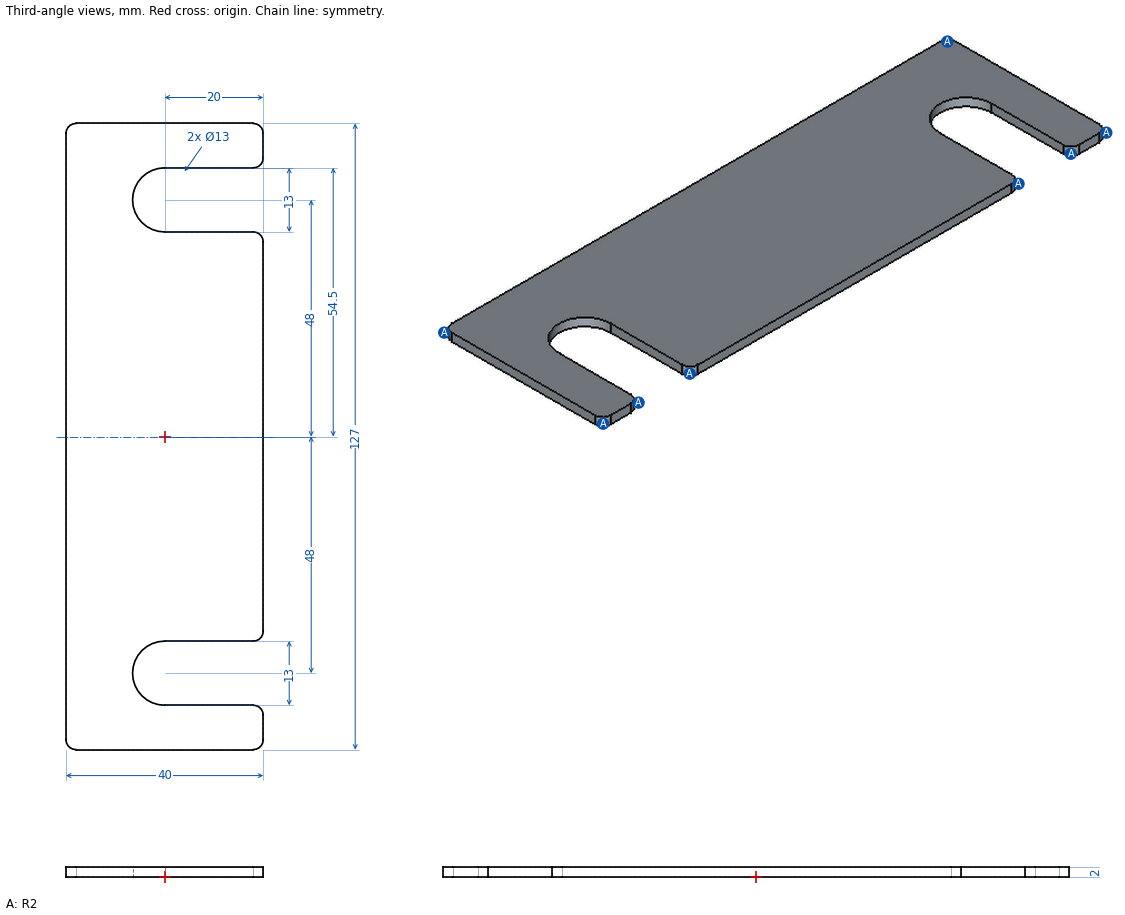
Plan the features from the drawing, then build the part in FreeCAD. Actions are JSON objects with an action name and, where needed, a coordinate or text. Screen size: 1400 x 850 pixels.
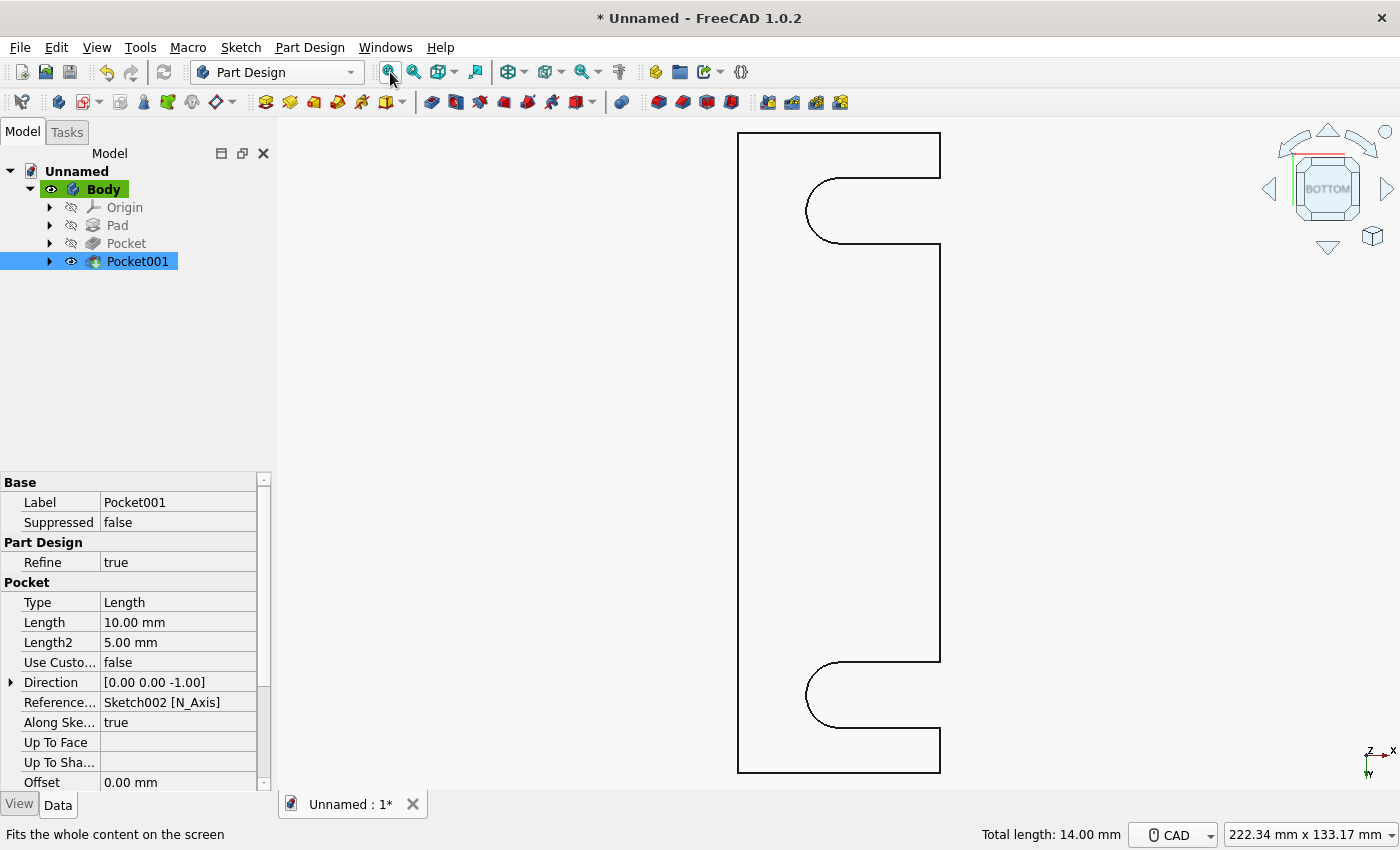
{"action": "key", "text": "4"}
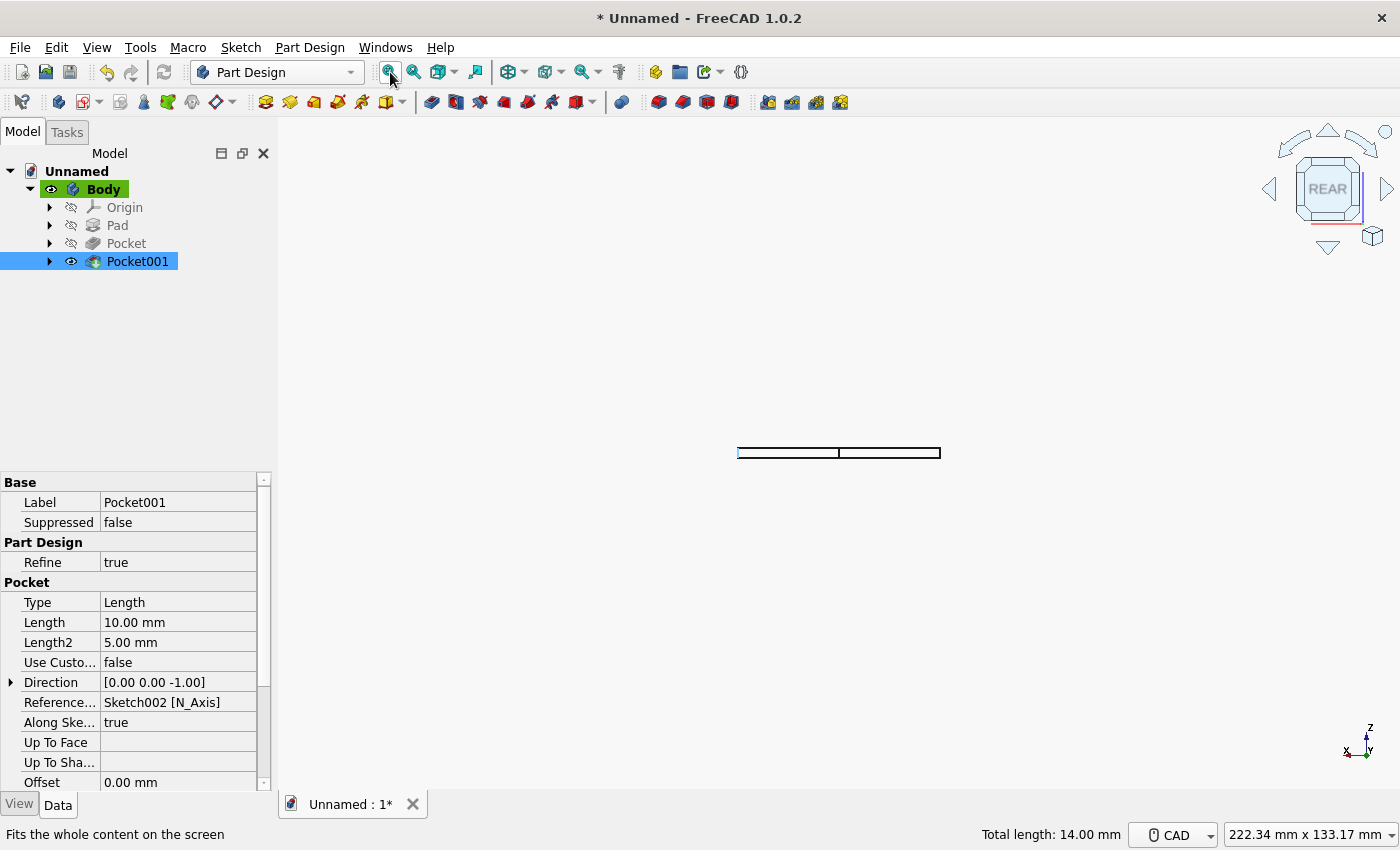
{"action": "key", "text": "v f"}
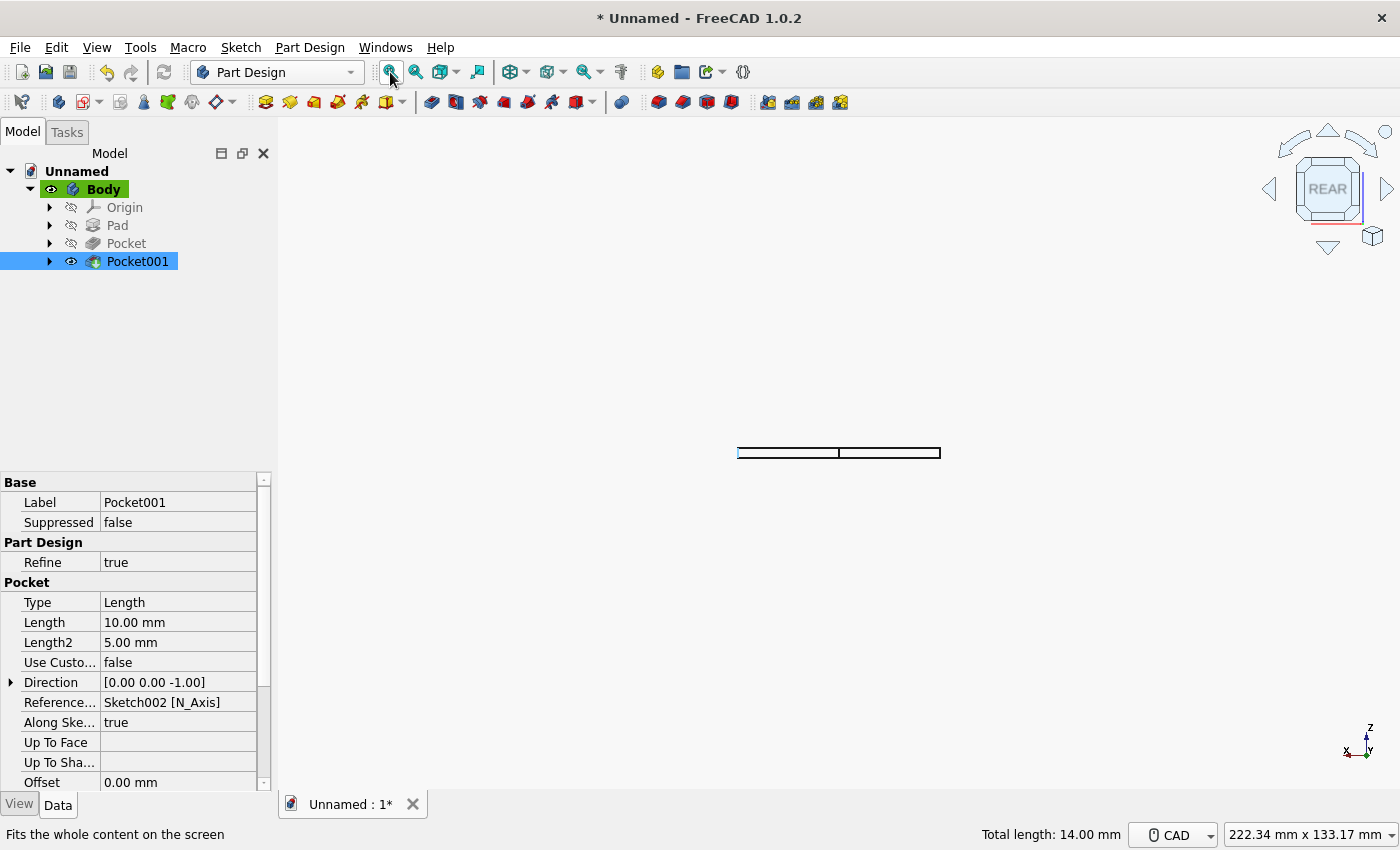
{"action": "left_click", "coordinate": [940, 452], "text": "ctrl"}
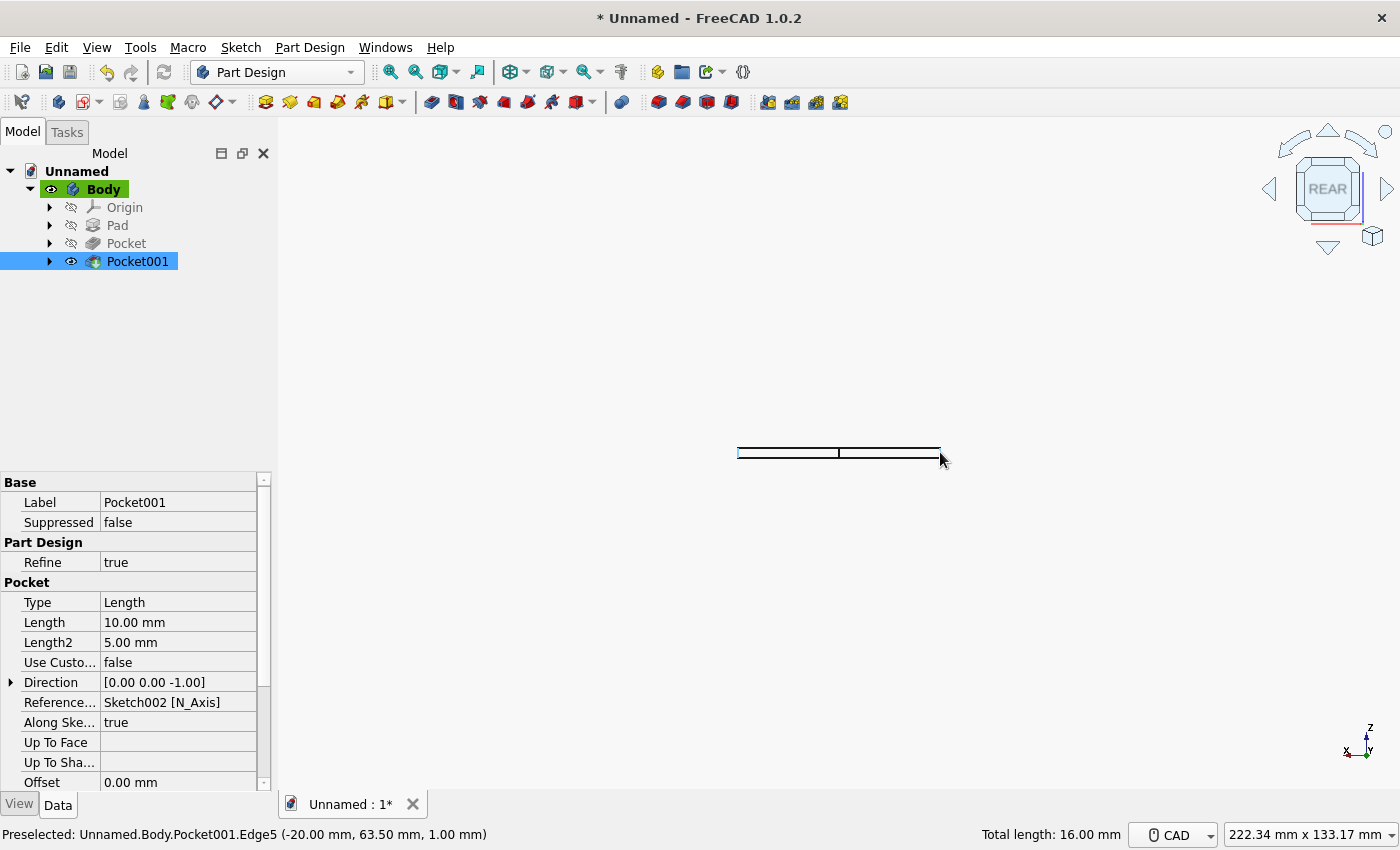
{"action": "key", "text": "v 1"}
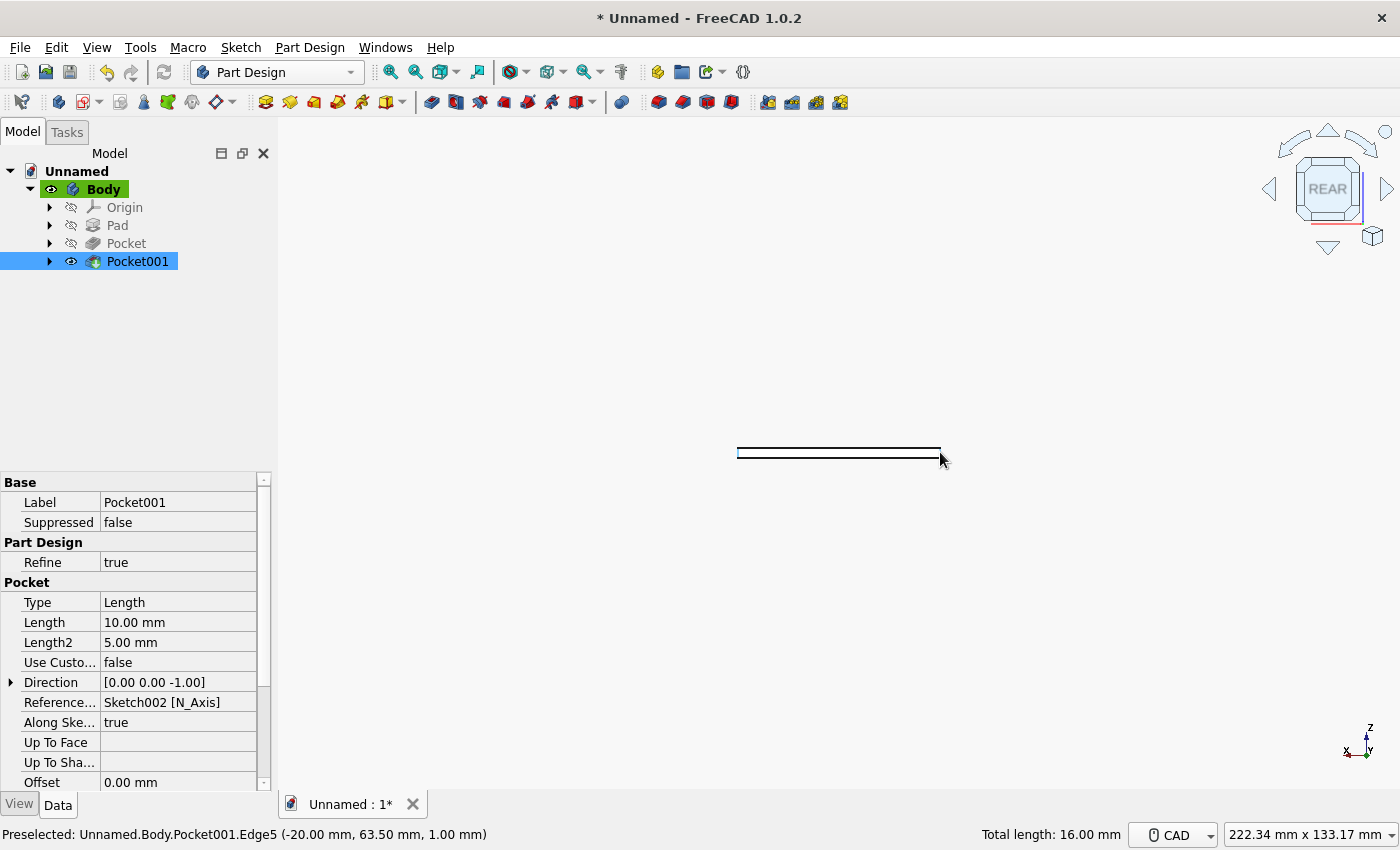
{"action": "left_click", "coordinate": [660, 102]}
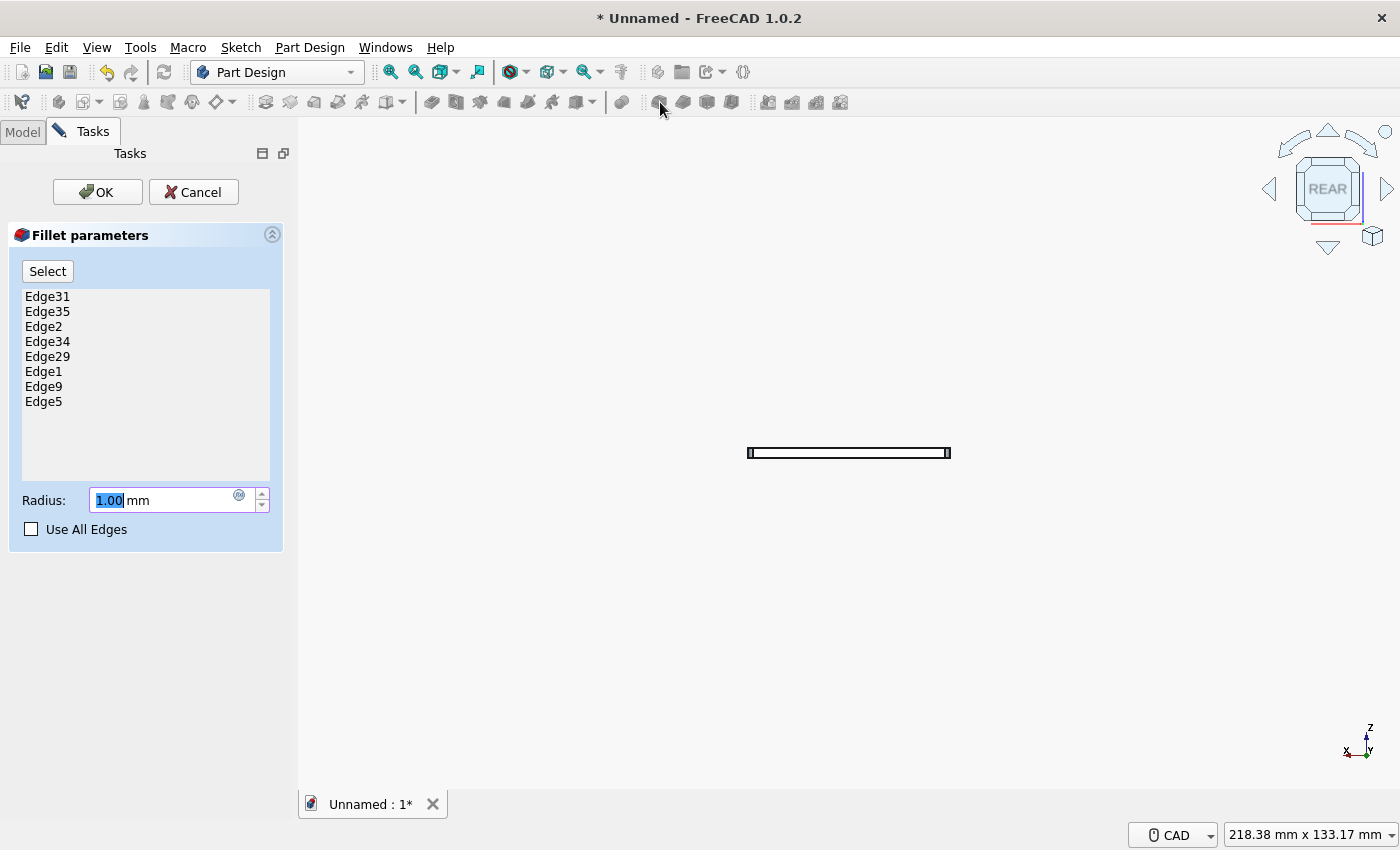
{"action": "type", "text": "2"}
{"action": "key", "text": "Tab"}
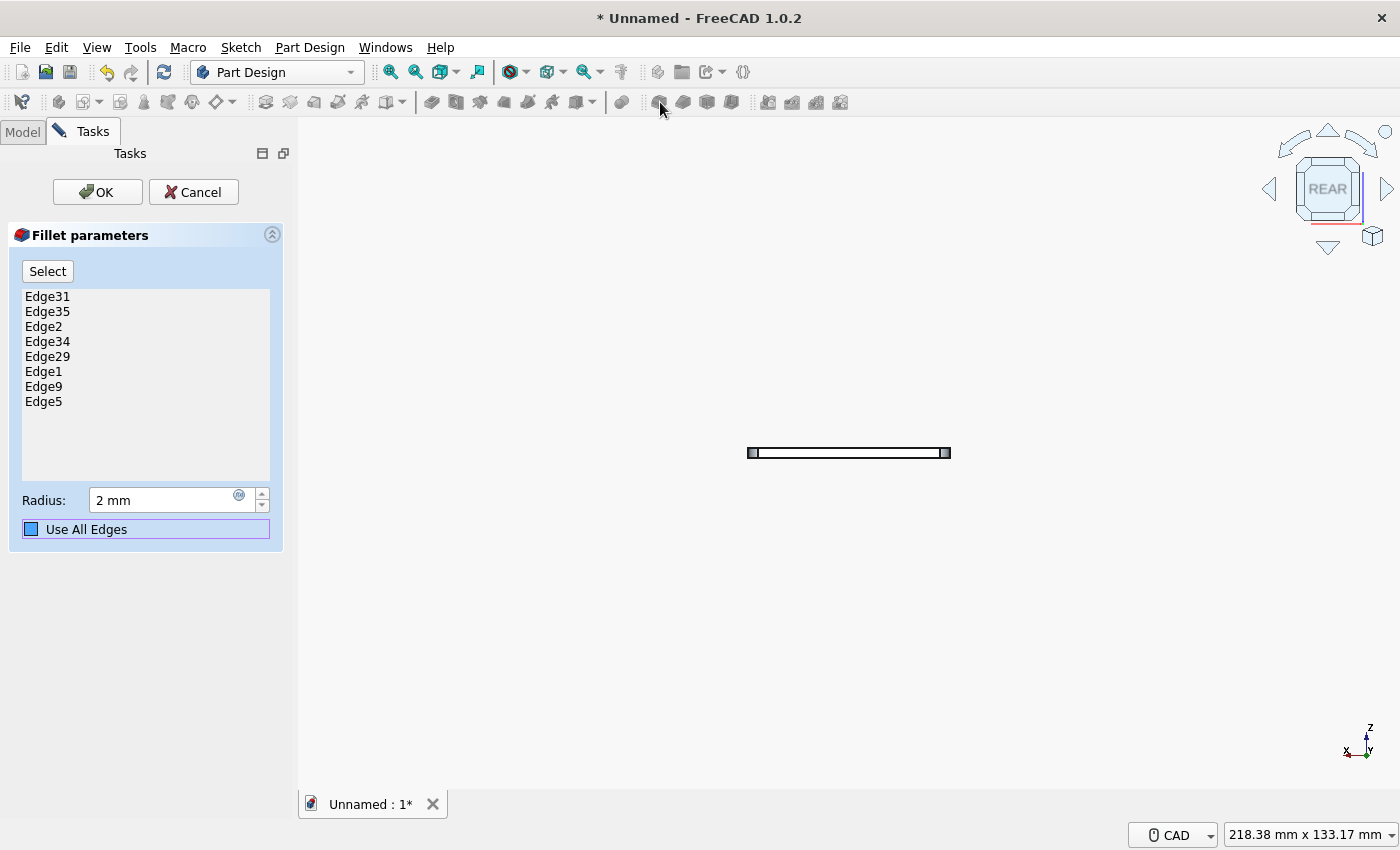
{"action": "left_click", "coordinate": [98, 192]}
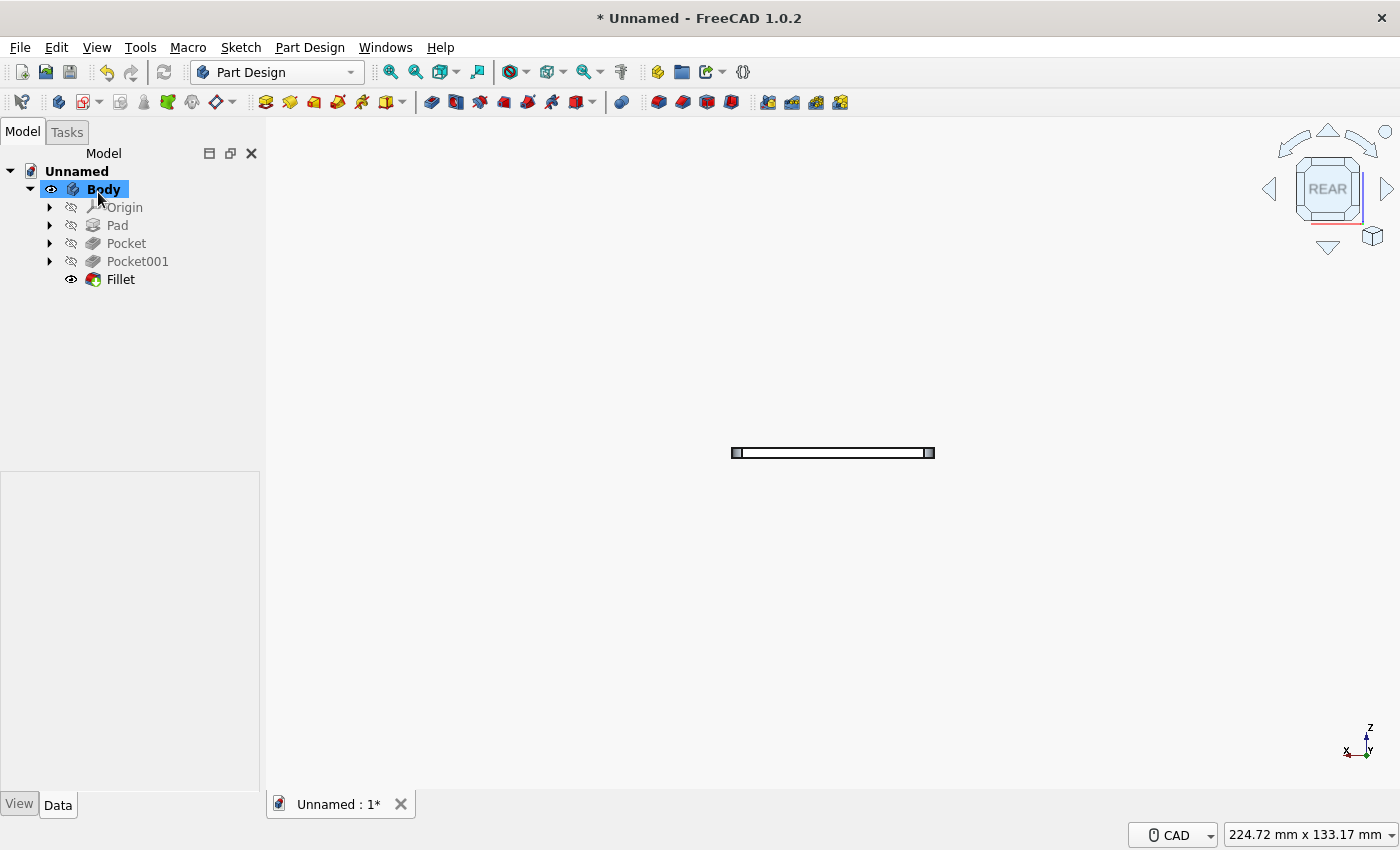
{"action": "key", "text": "0"}